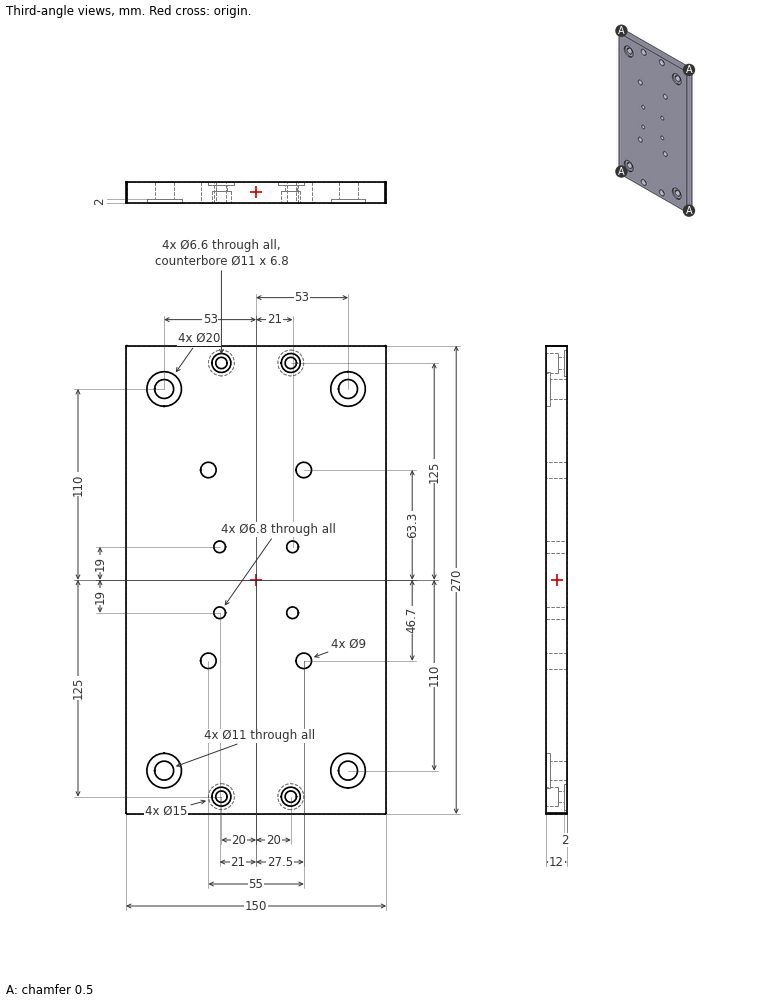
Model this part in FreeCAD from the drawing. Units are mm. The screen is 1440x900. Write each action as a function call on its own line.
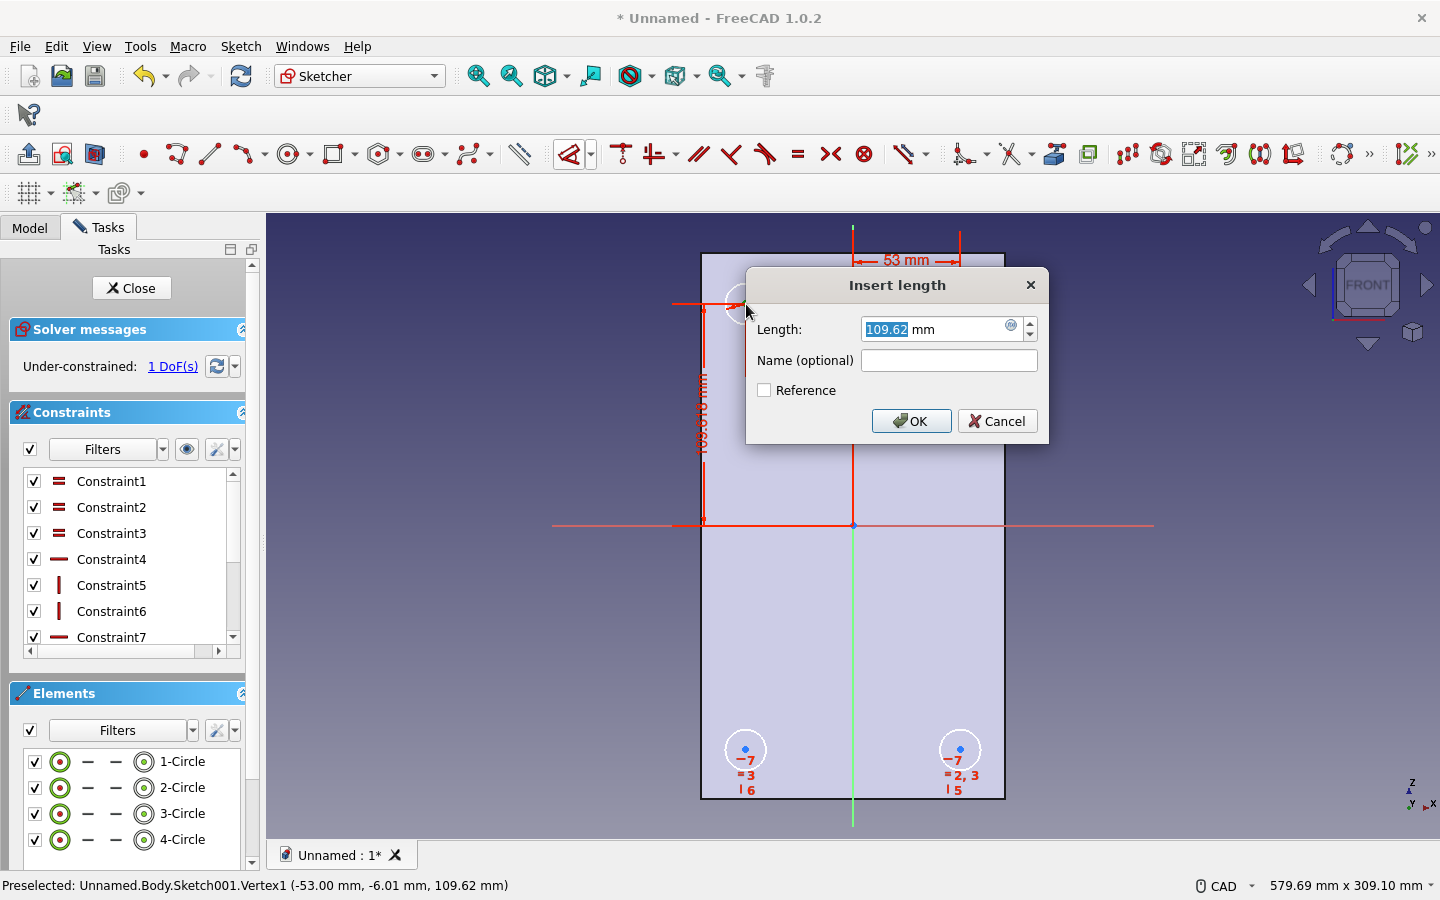
text(110)
key(Return)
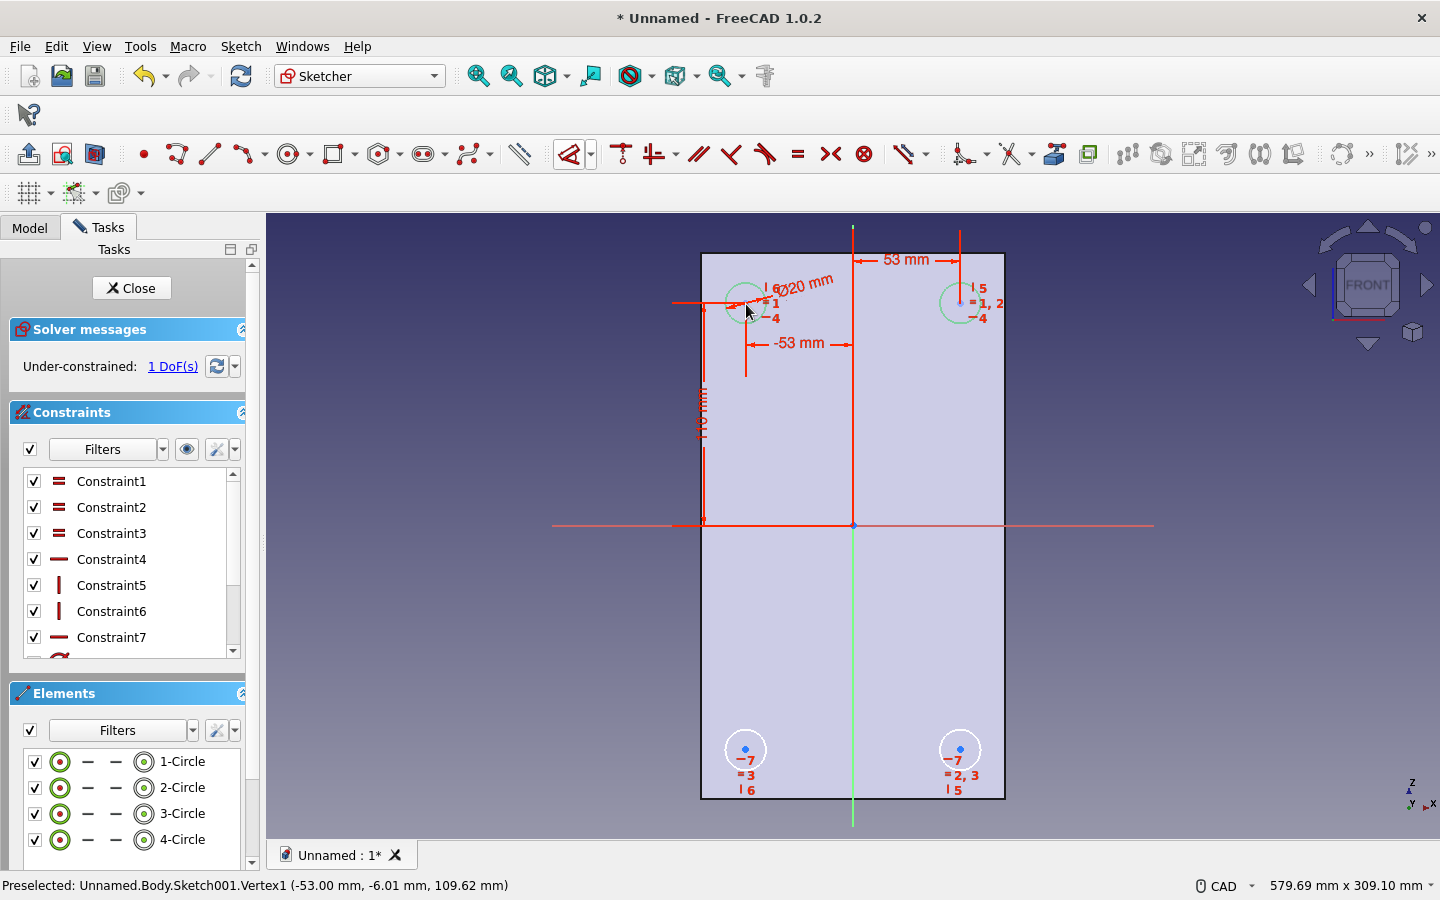
click(960, 750)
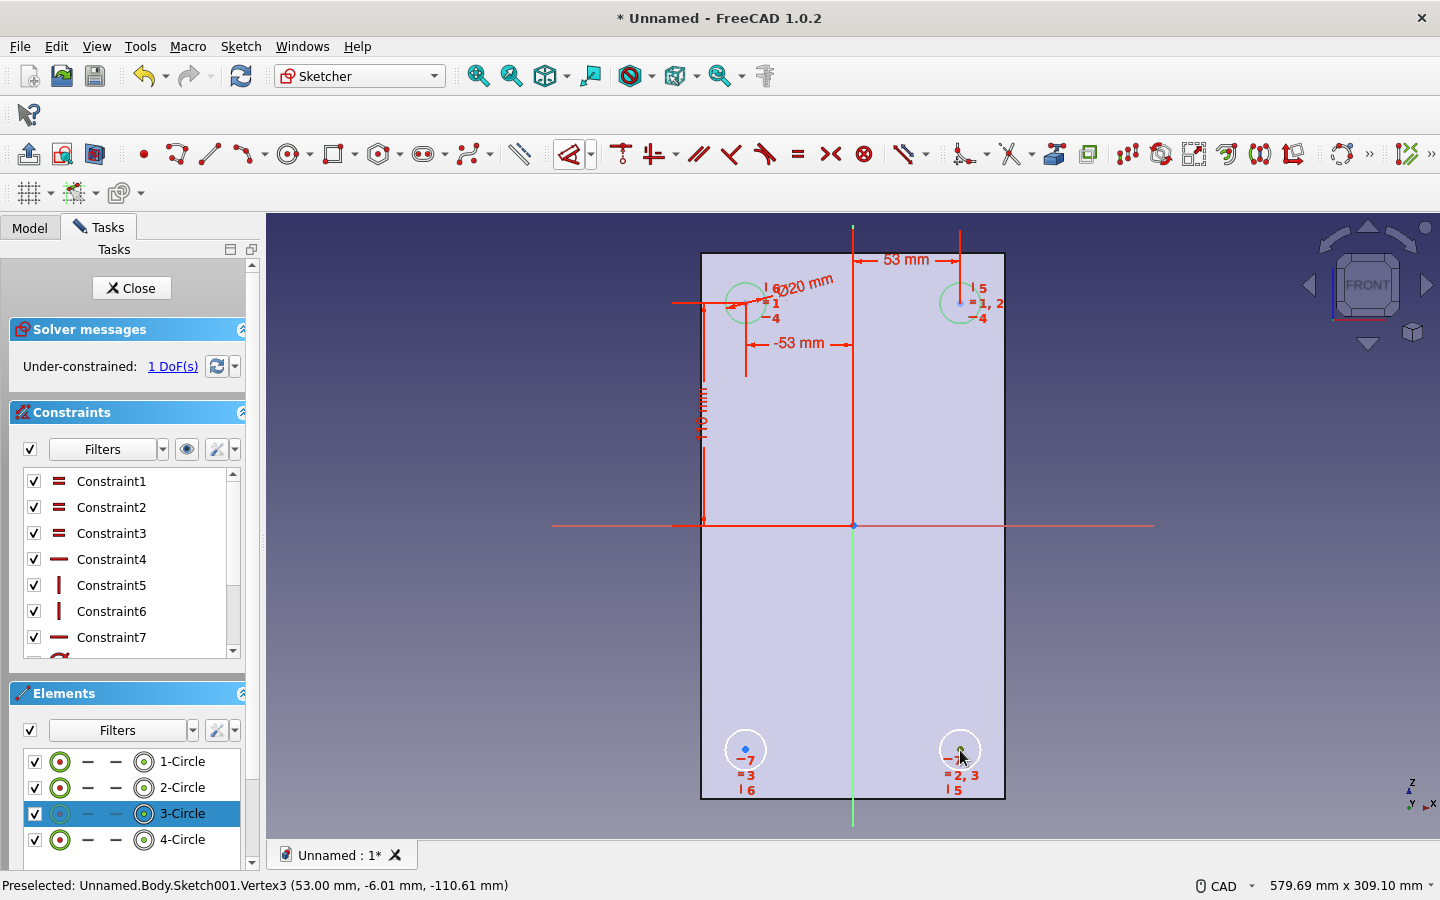
key(i)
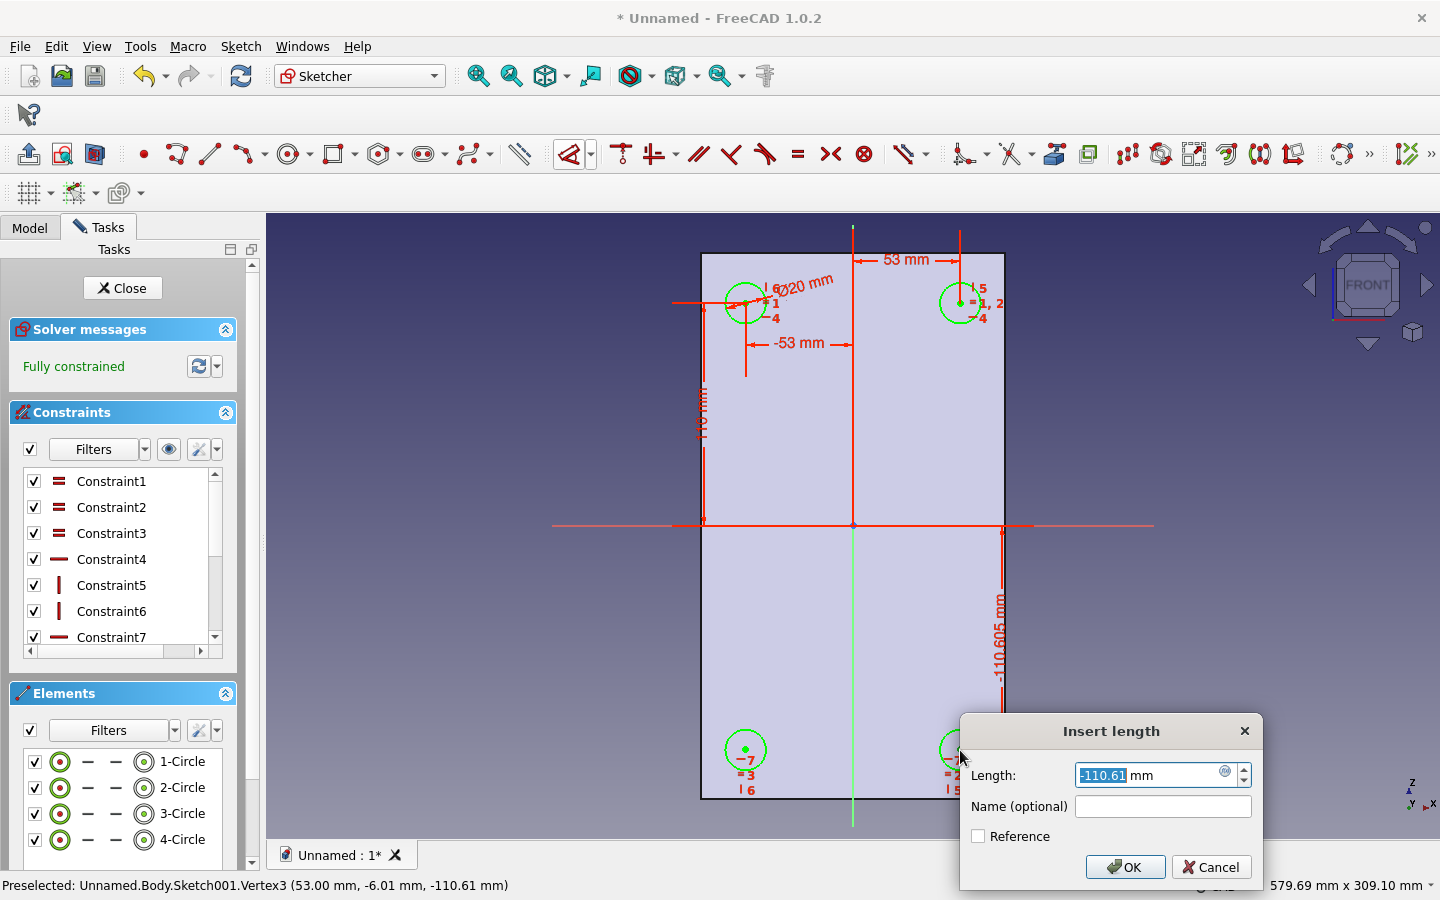
text(-110)
key(Return)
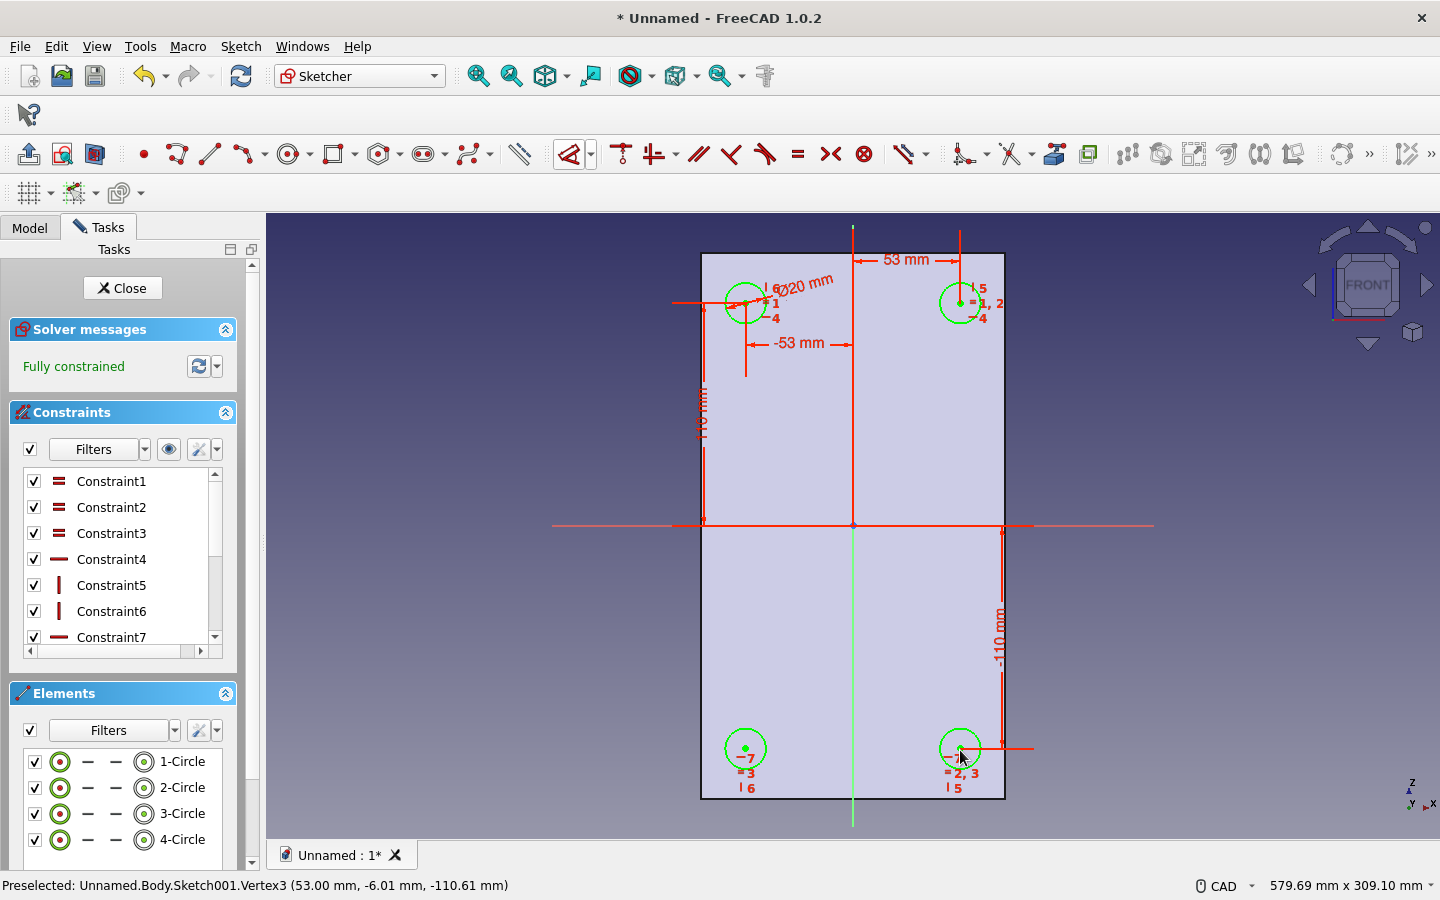
click(123, 288)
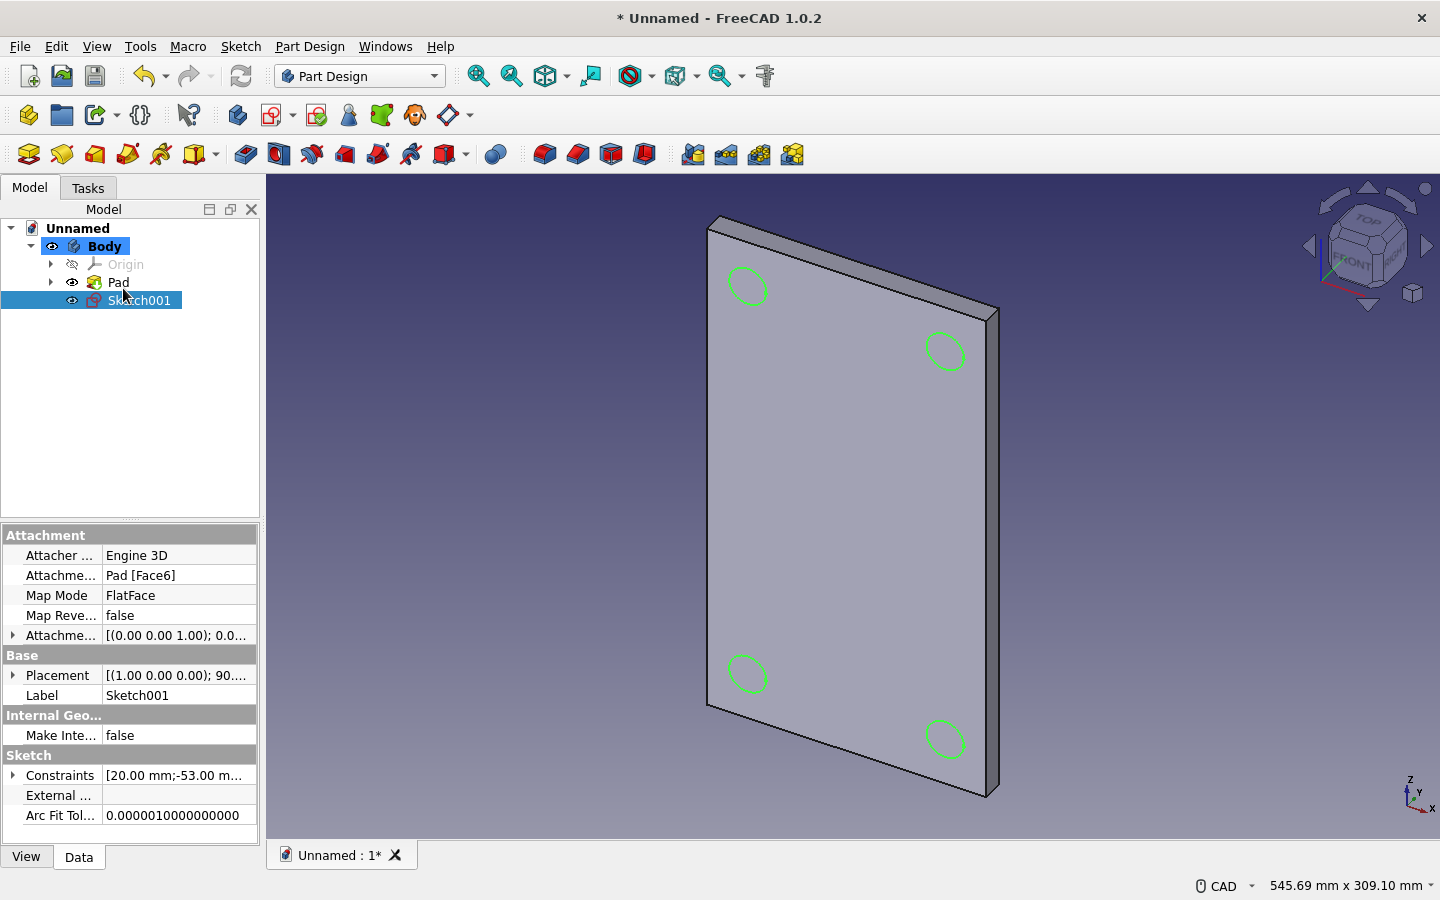
click(246, 154)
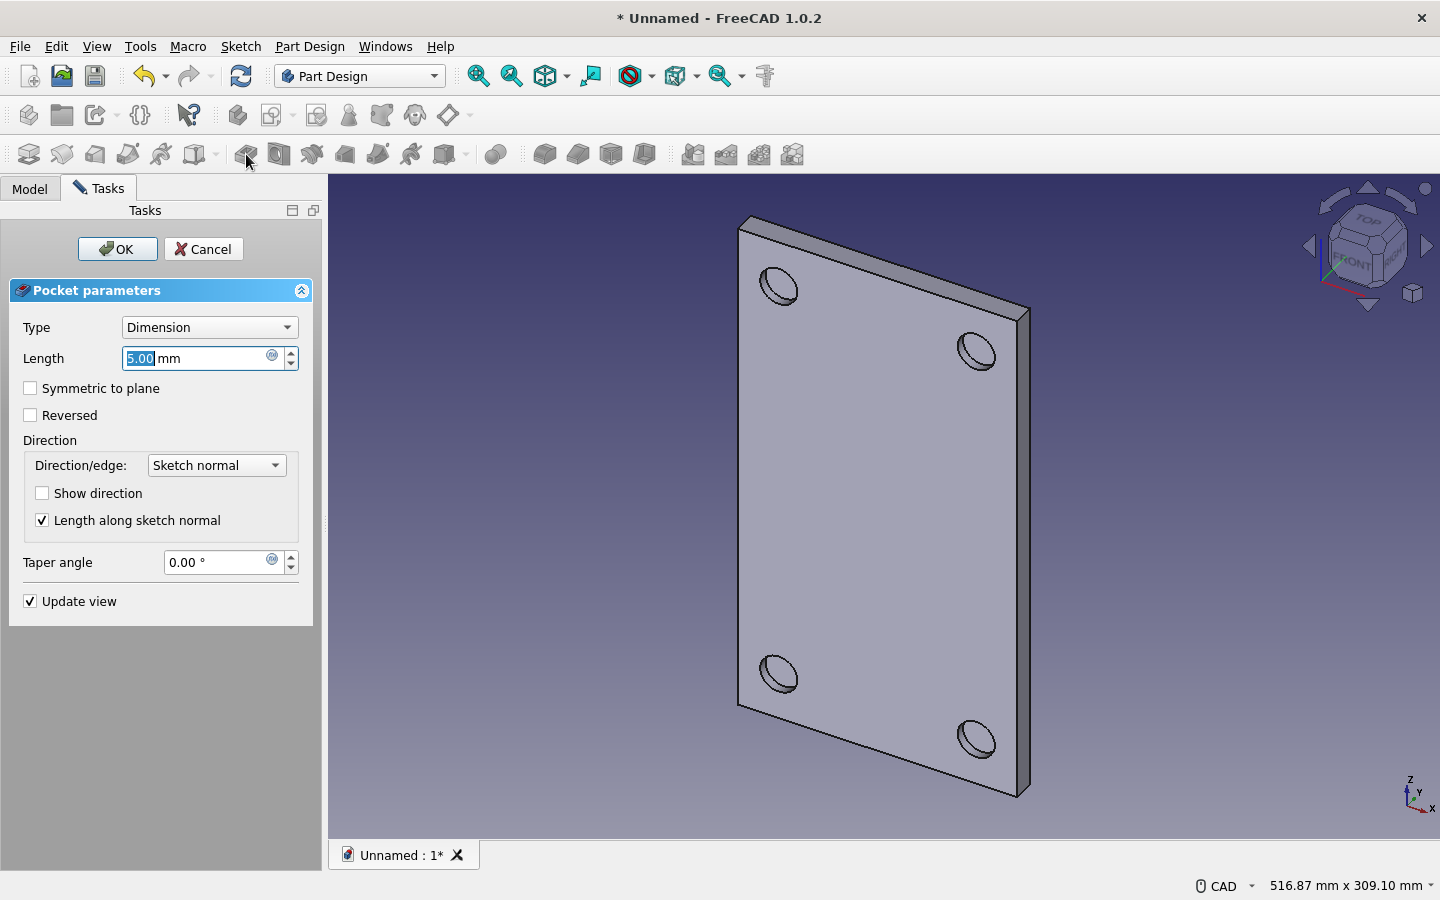
text(2)
key(Tab)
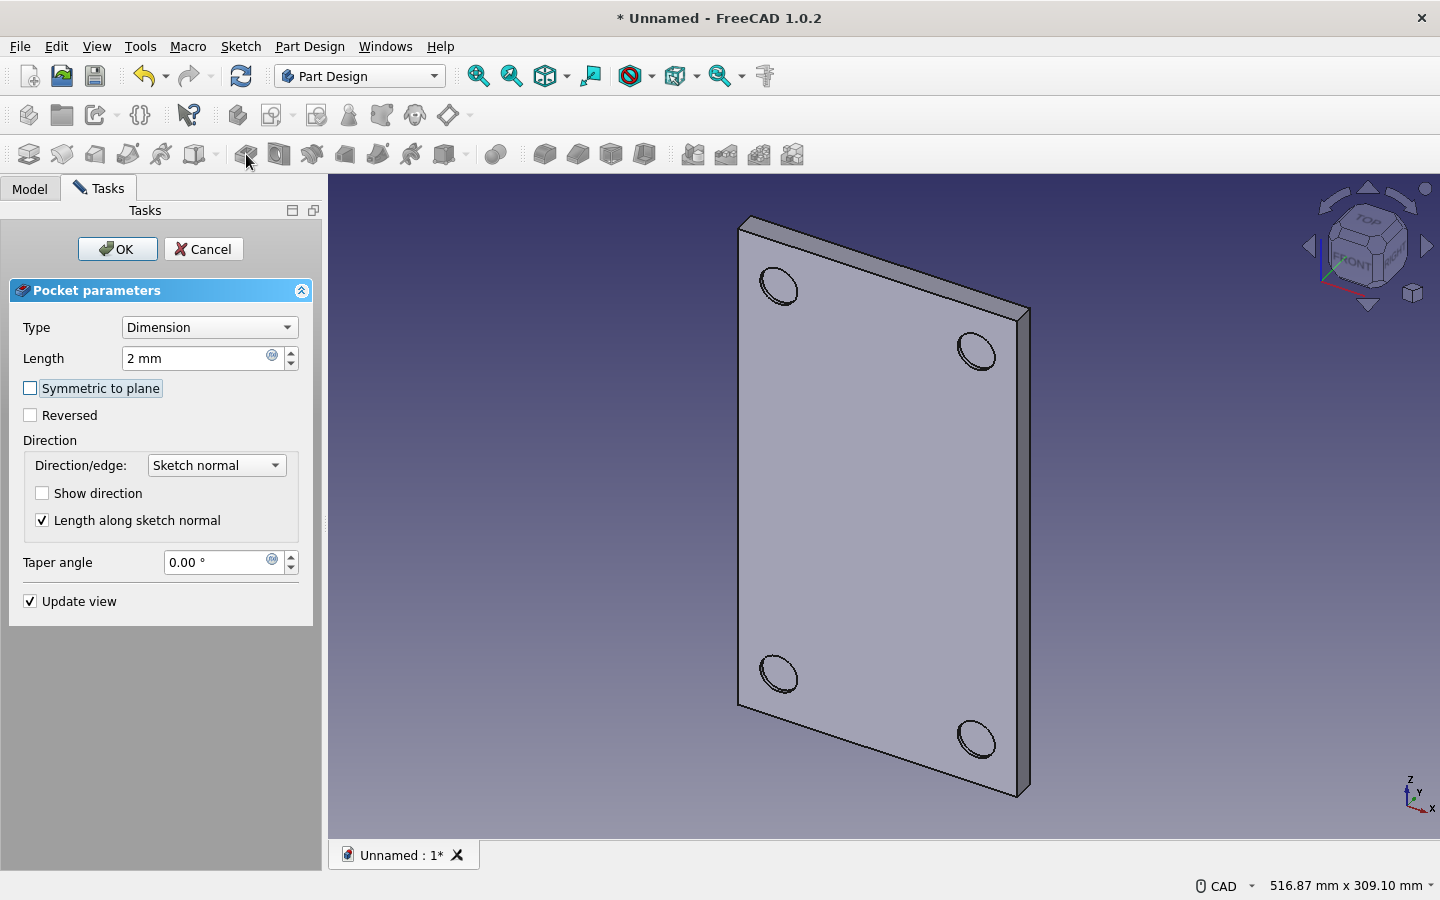
click(118, 249)